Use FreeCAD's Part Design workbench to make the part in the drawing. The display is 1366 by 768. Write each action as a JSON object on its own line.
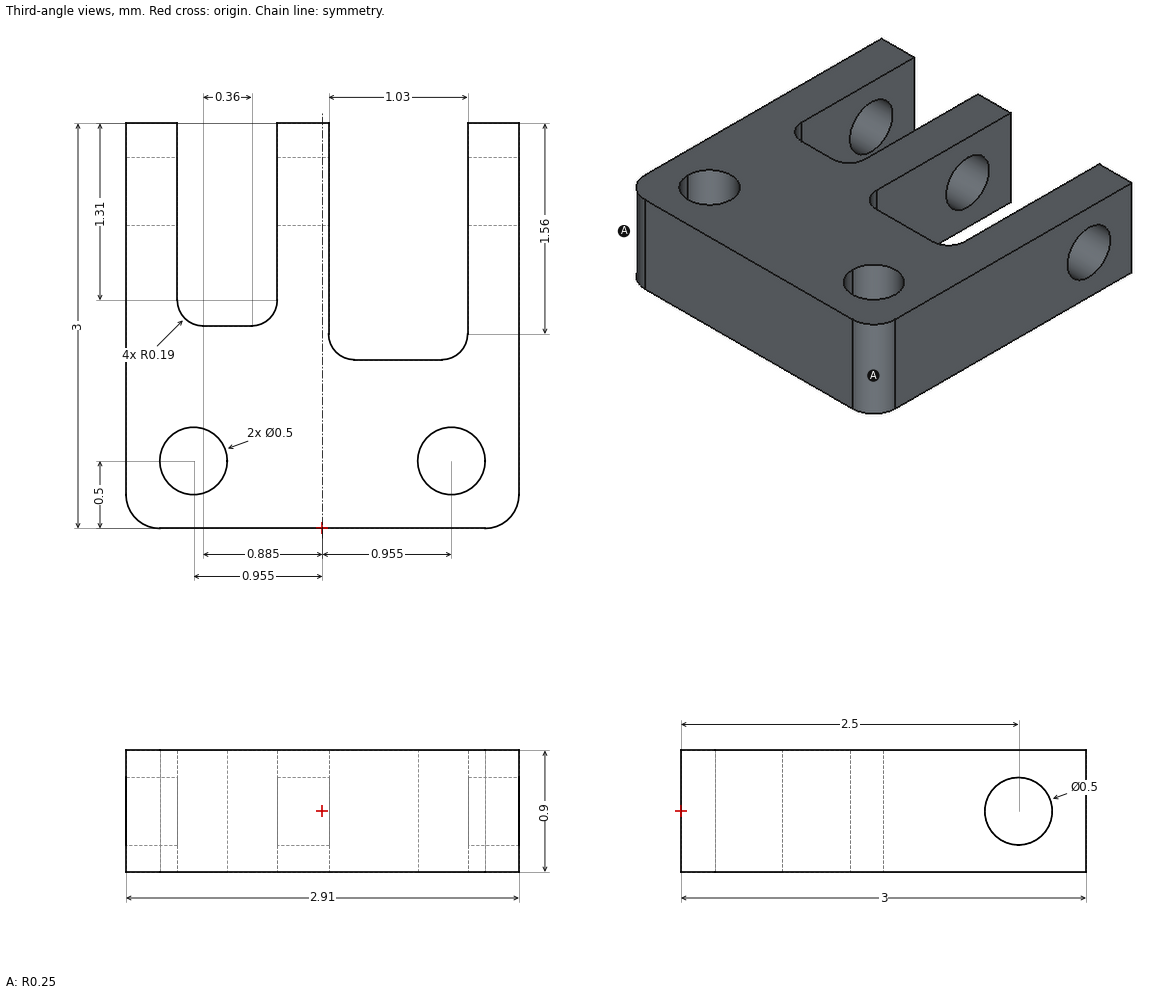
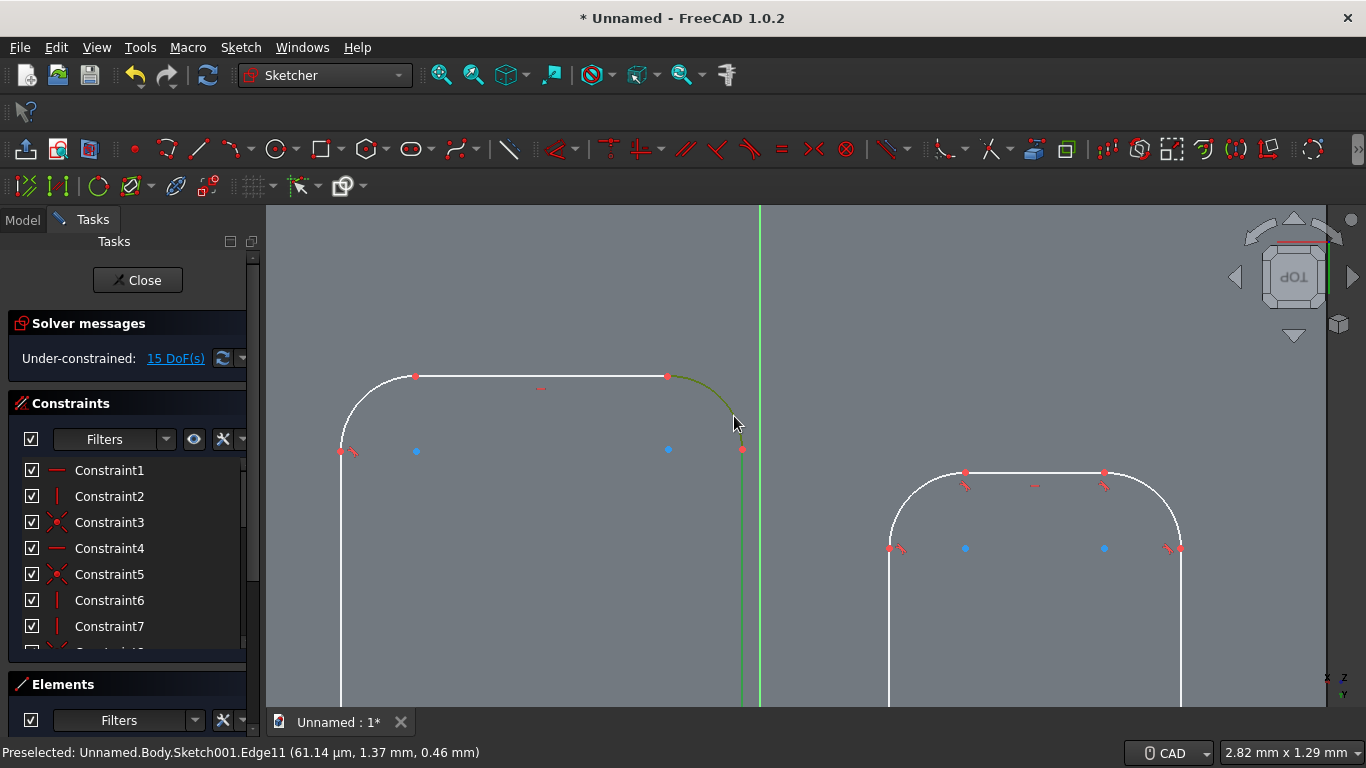
{"action": "key", "text": "t"}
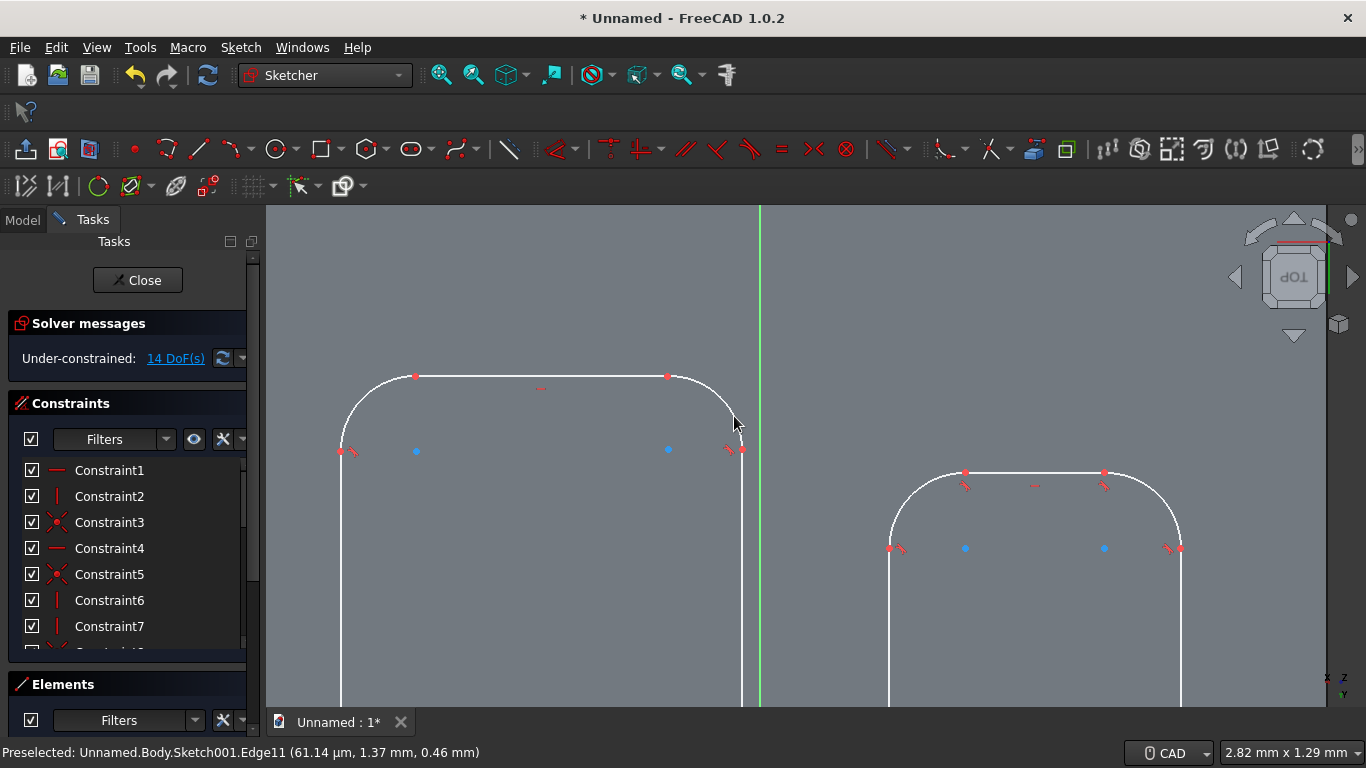
{"action": "left_click", "coordinate": [592, 376]}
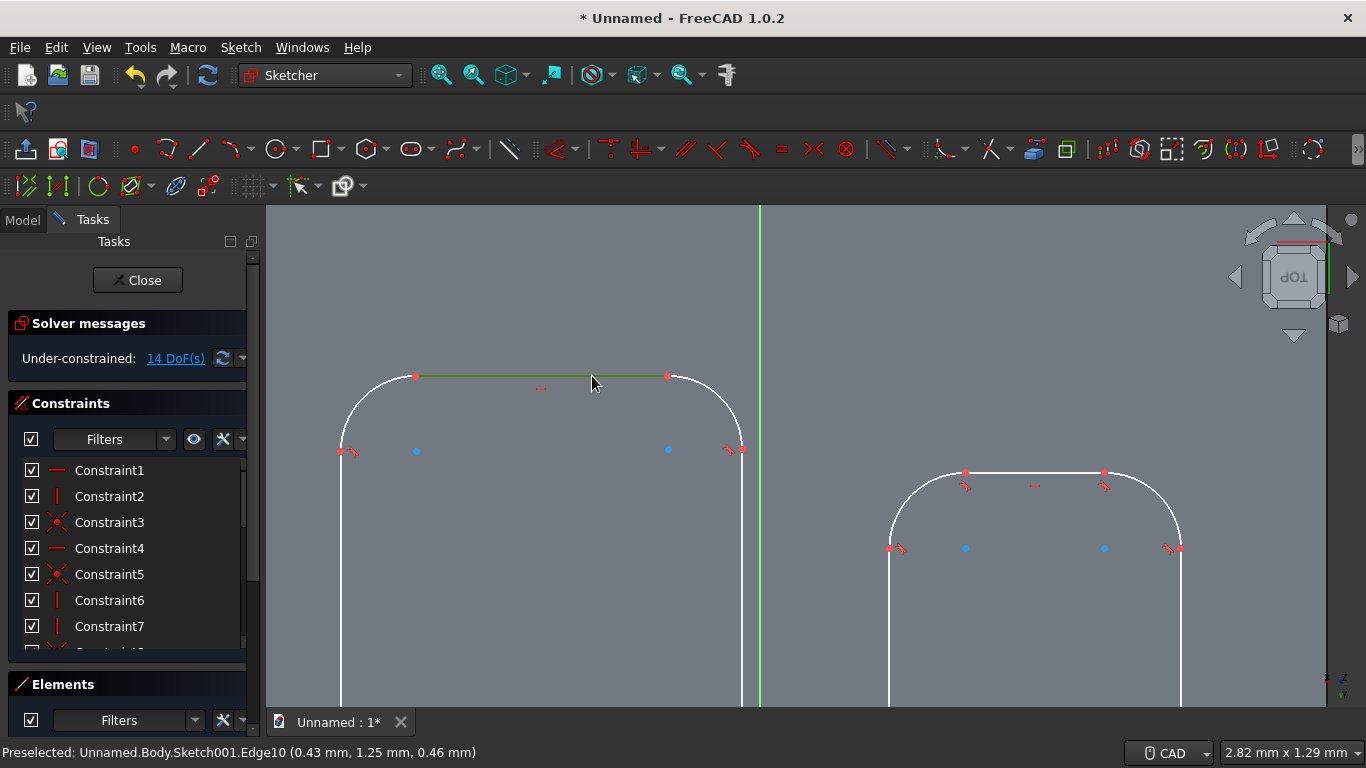
{"action": "left_click", "coordinate": [734, 416]}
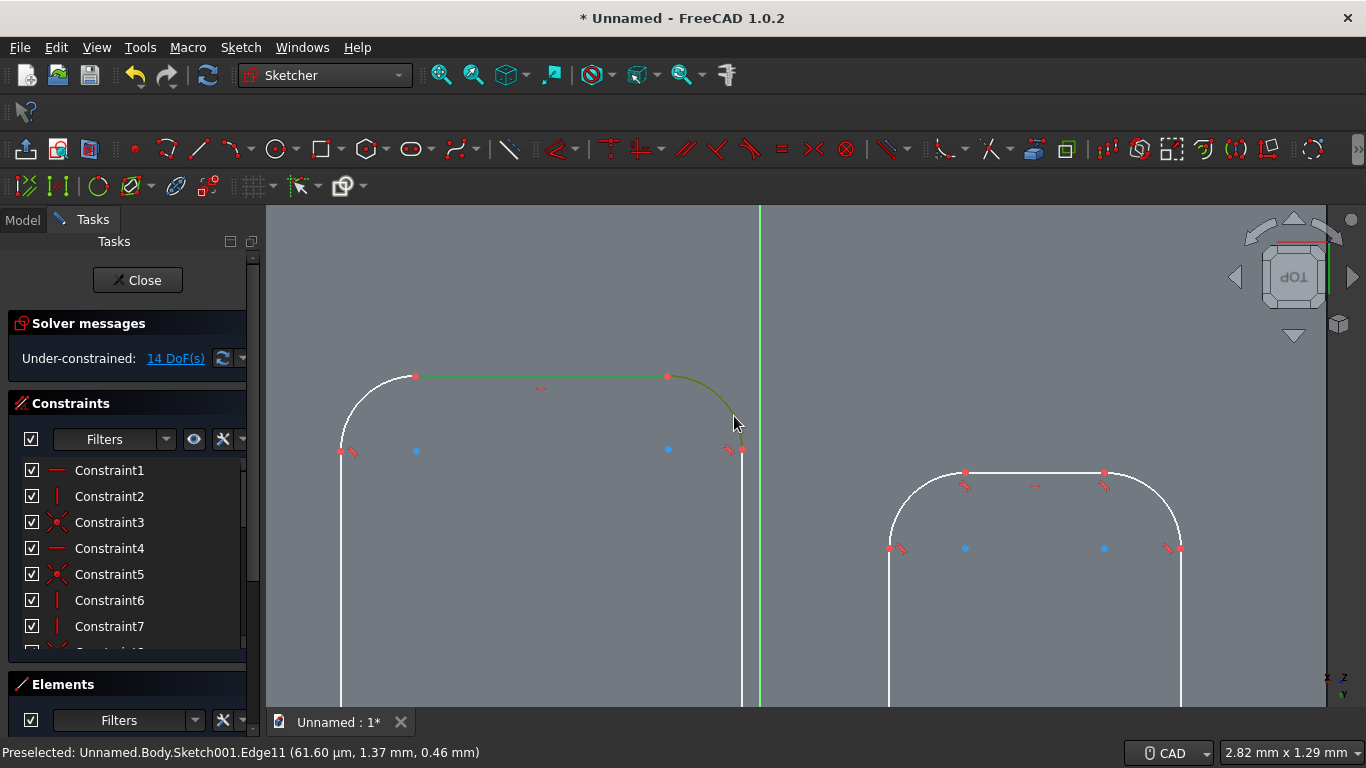
{"action": "left_click", "coordinate": [750, 150]}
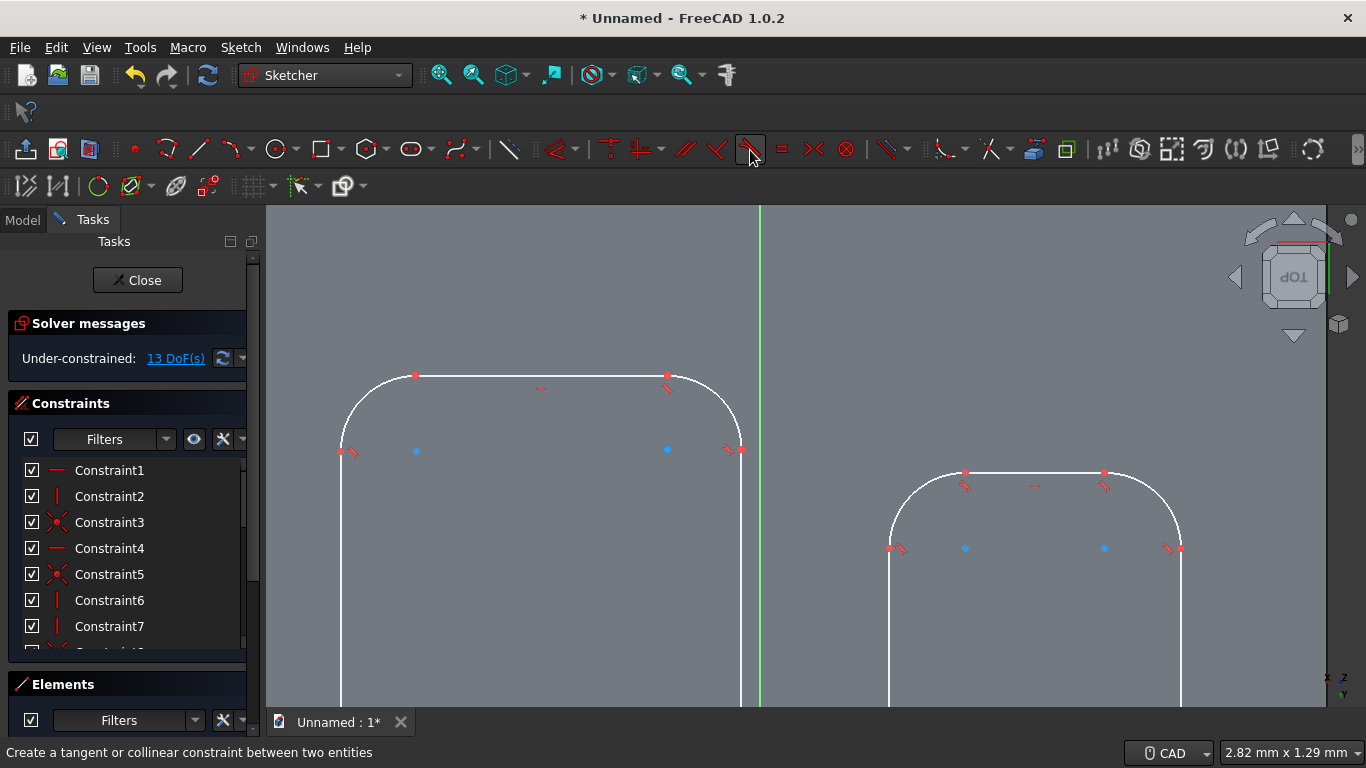
{"action": "left_click", "coordinate": [592, 376]}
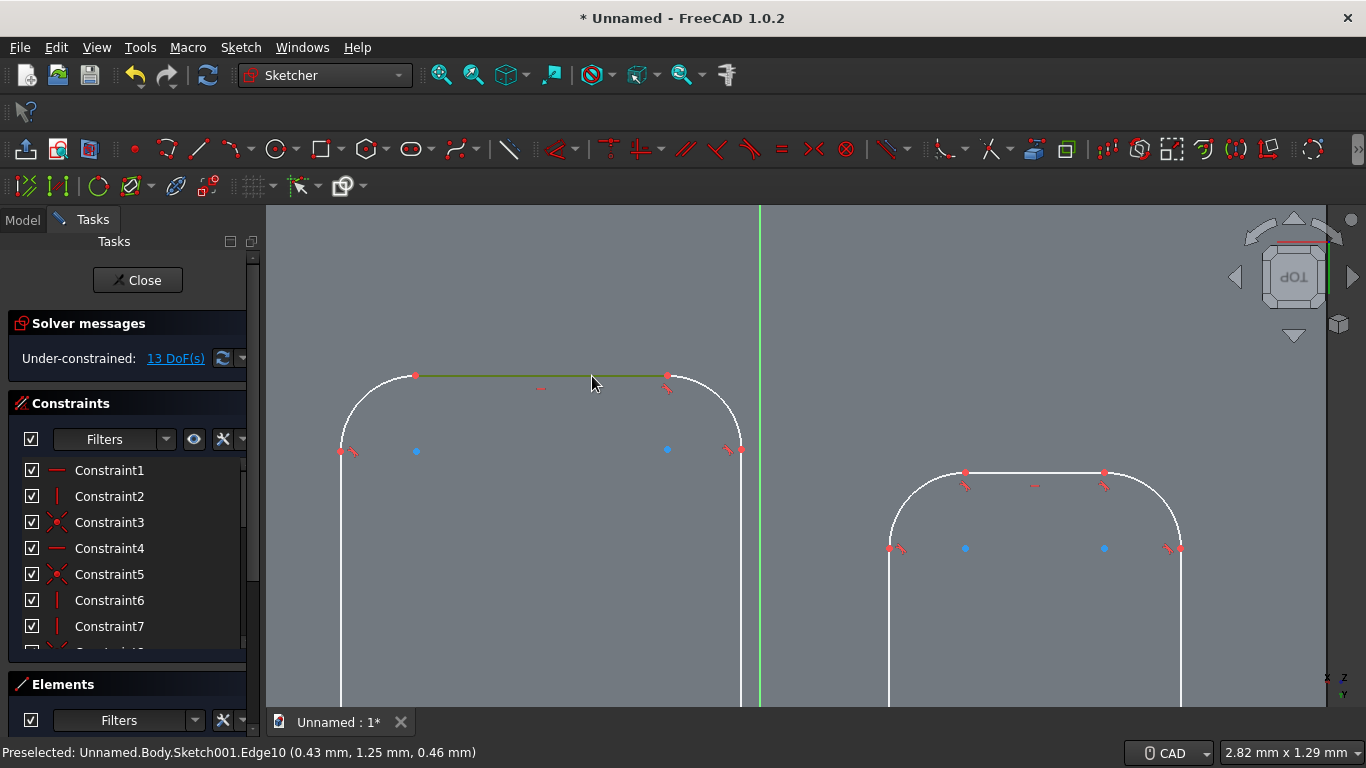
{"action": "left_click", "coordinate": [381, 385]}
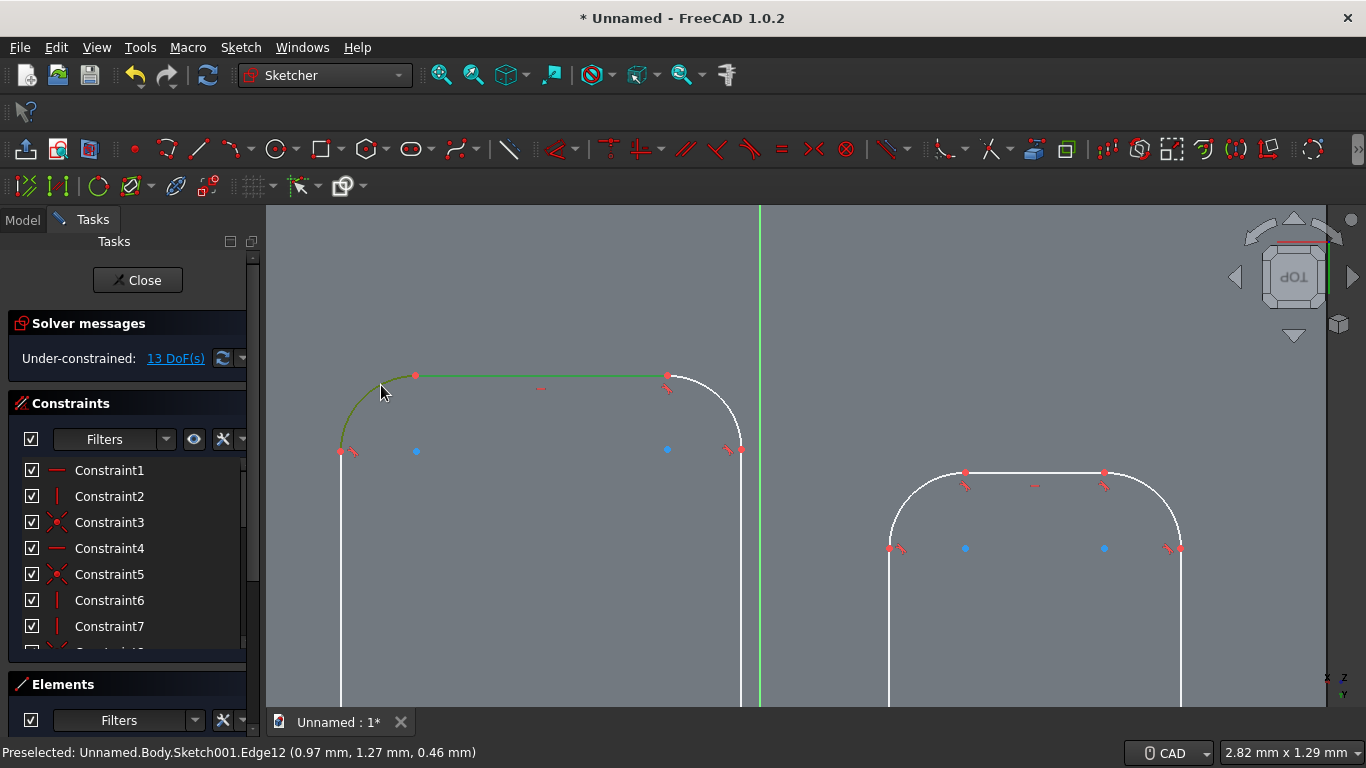
{"action": "key", "text": "t"}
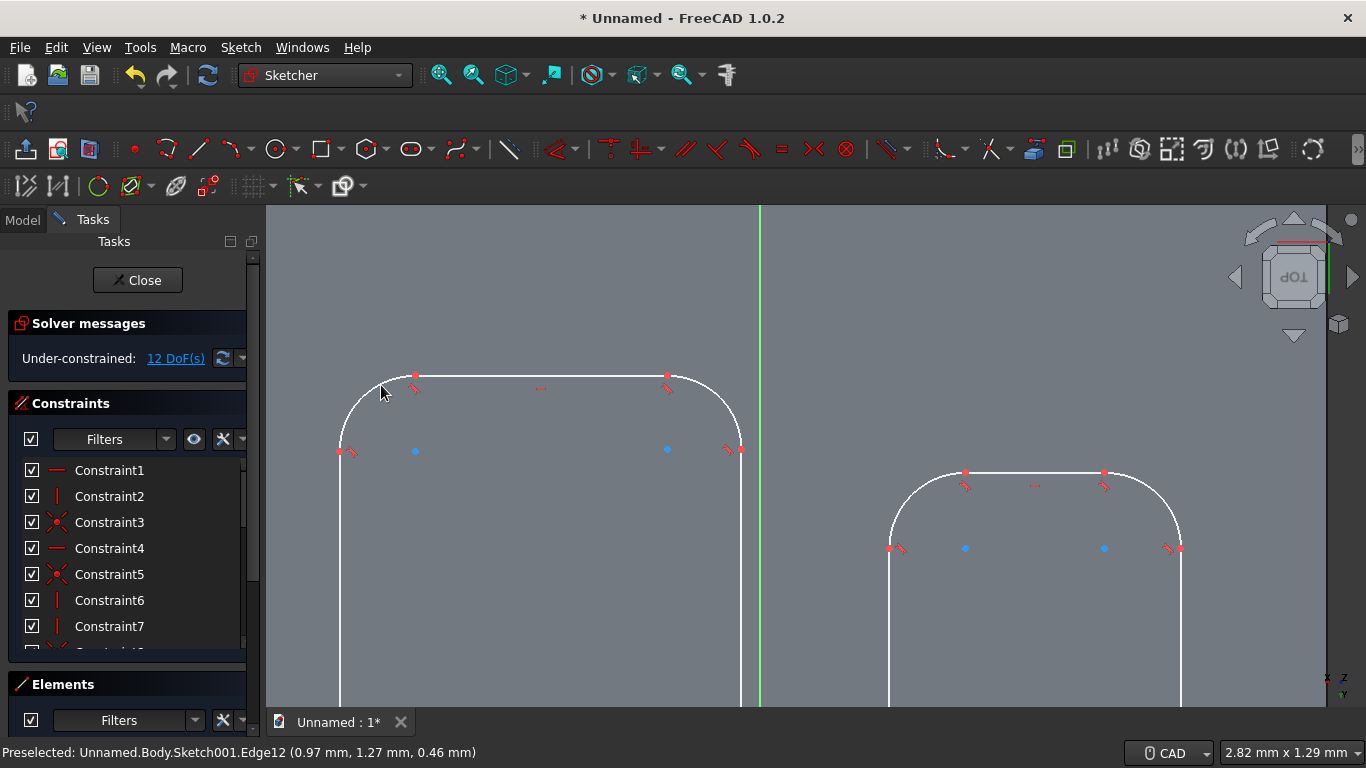
{"action": "left_click", "coordinate": [931, 481]}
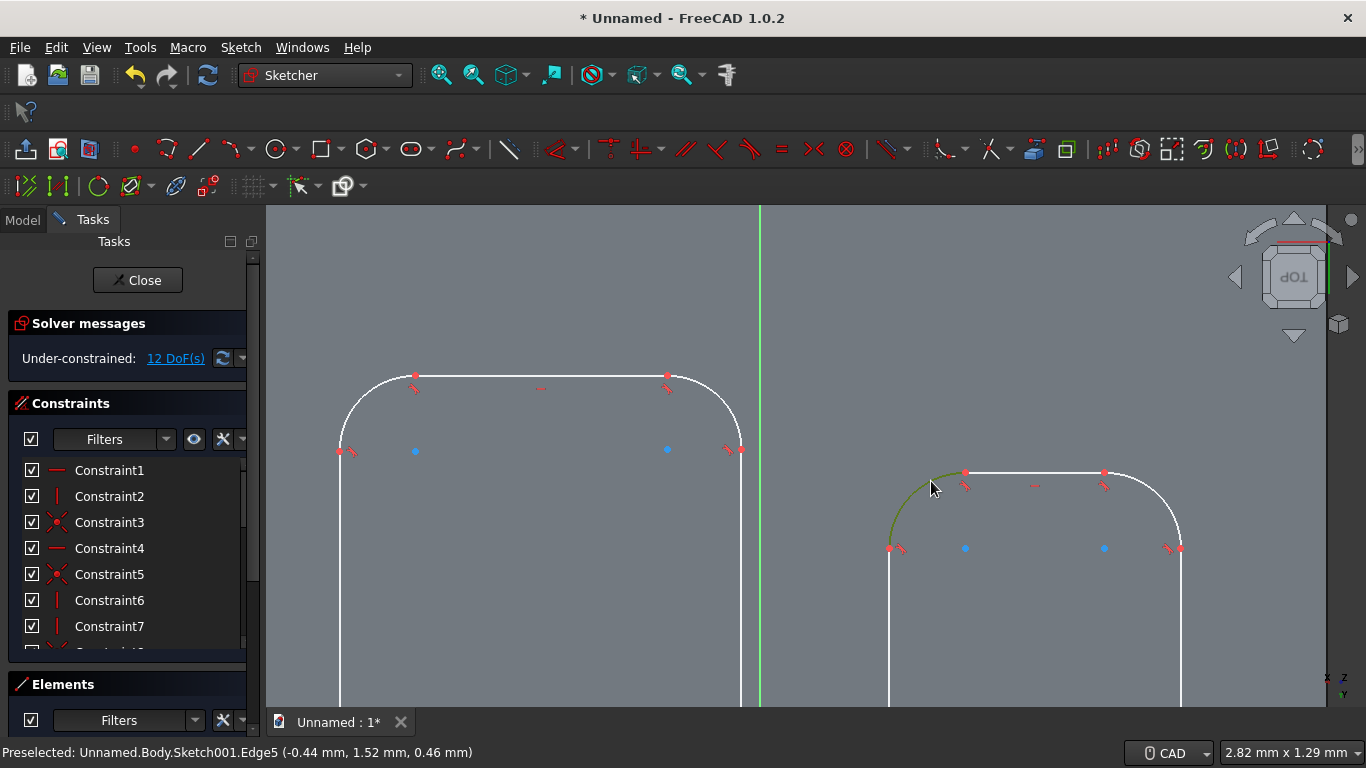
{"action": "left_click", "coordinate": [1173, 514]}